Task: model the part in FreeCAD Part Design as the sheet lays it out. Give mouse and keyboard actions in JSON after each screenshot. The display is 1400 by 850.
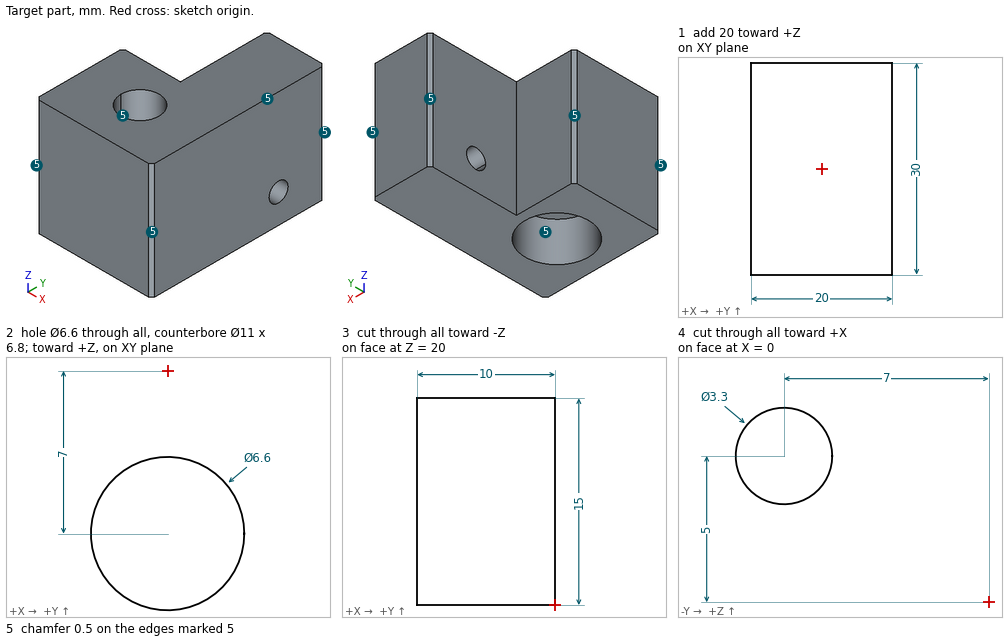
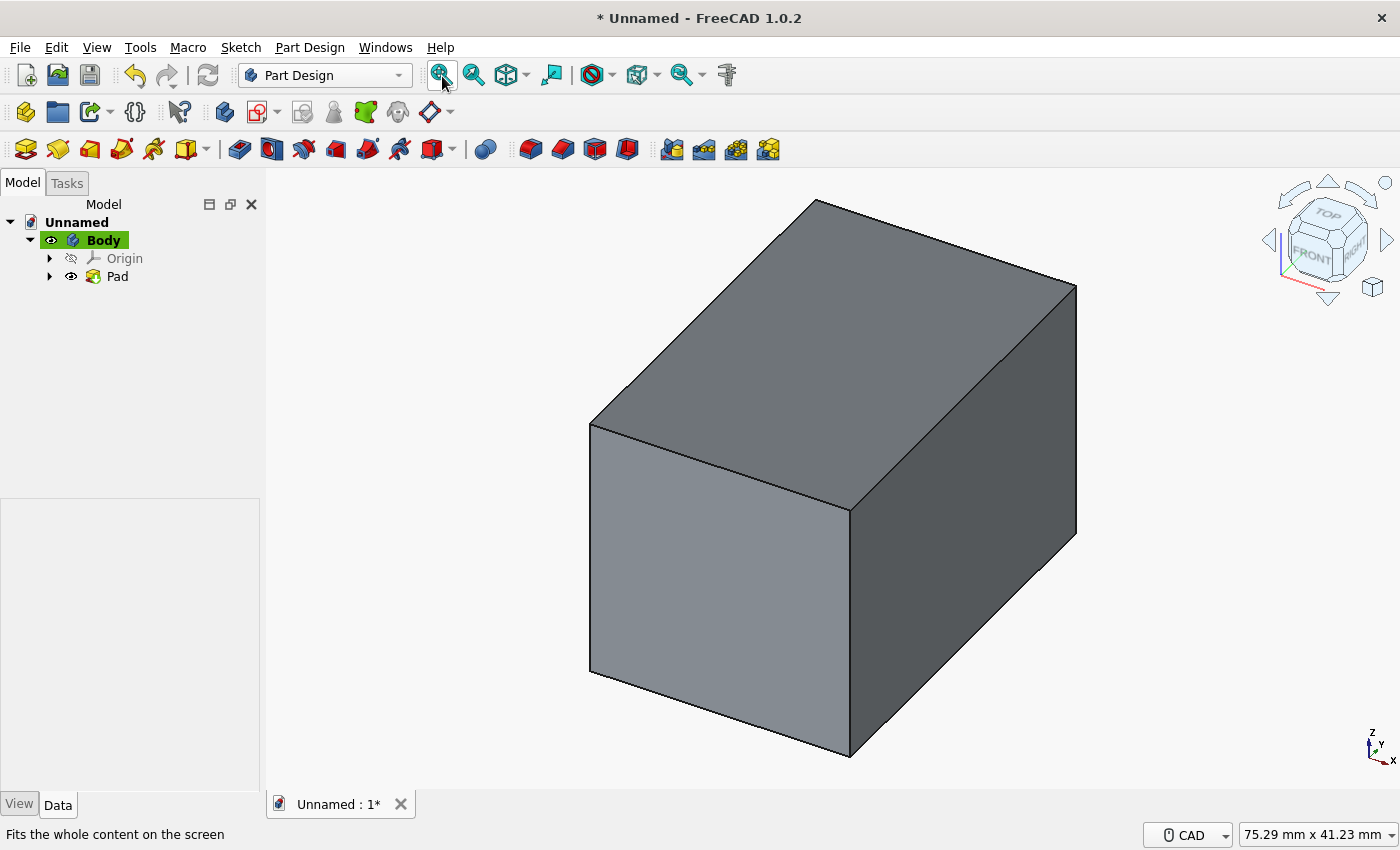
{"action": "left_click", "coordinate": [258, 112]}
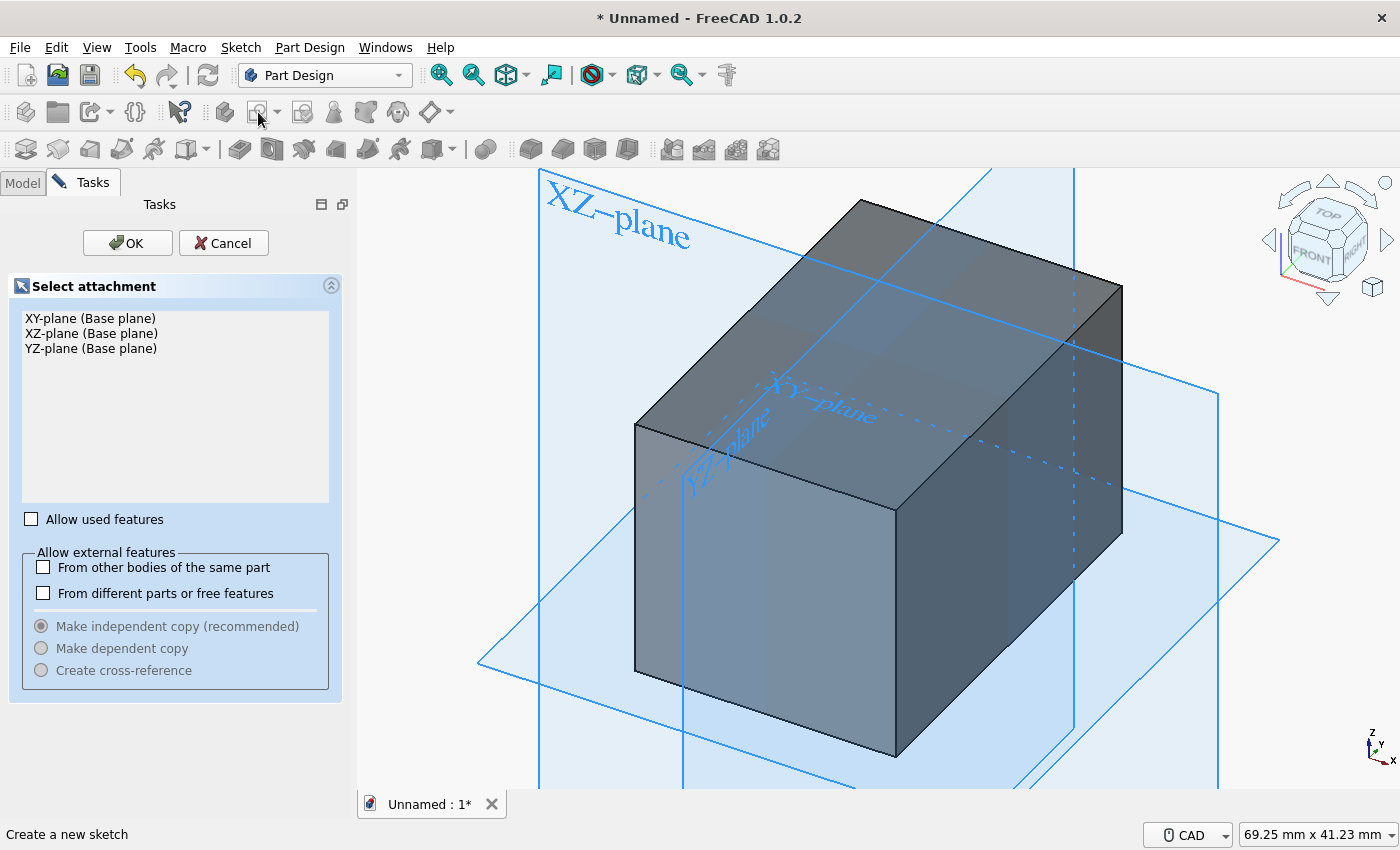
{"action": "left_click", "coordinate": [82, 318]}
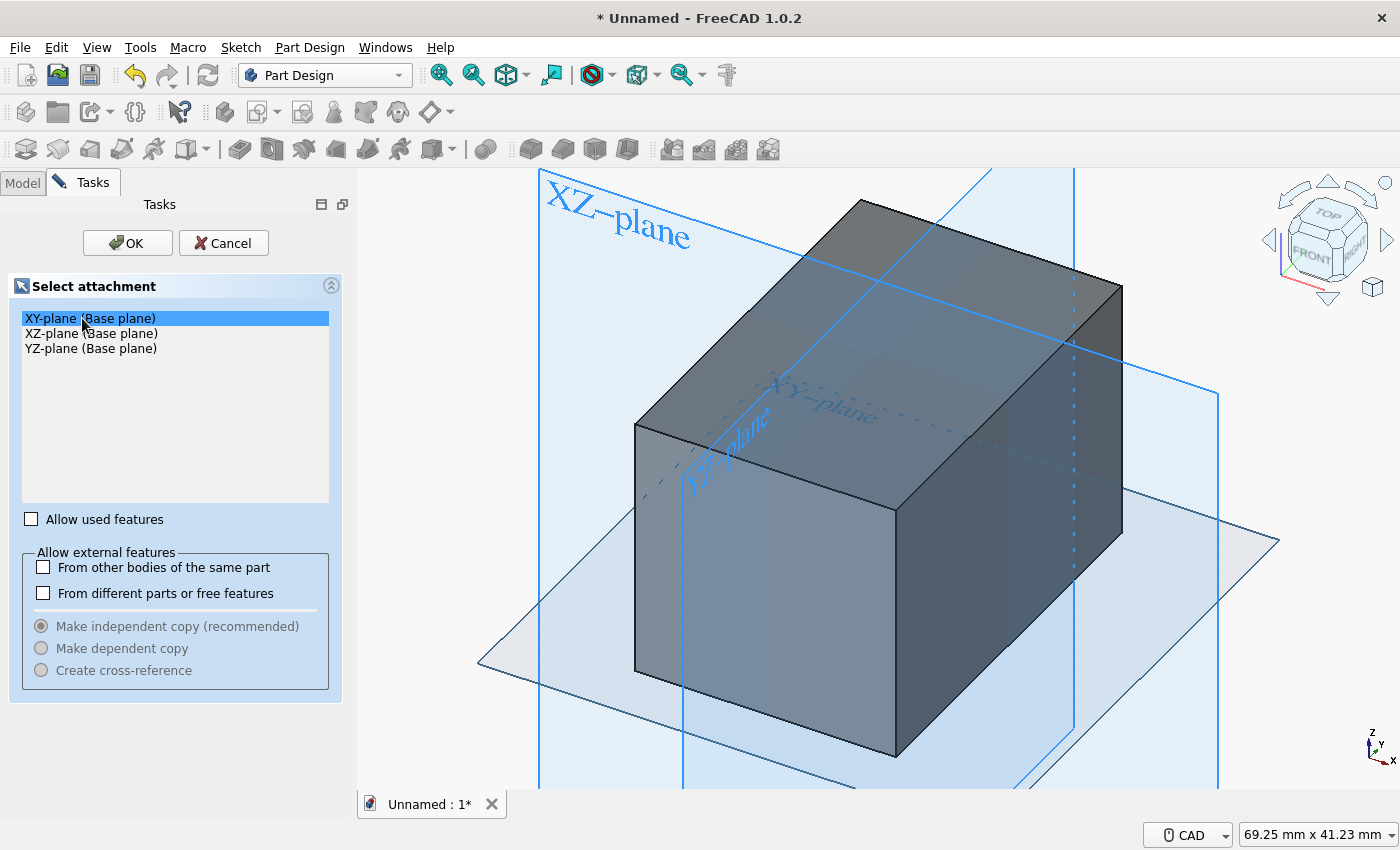
{"action": "left_click", "coordinate": [128, 243]}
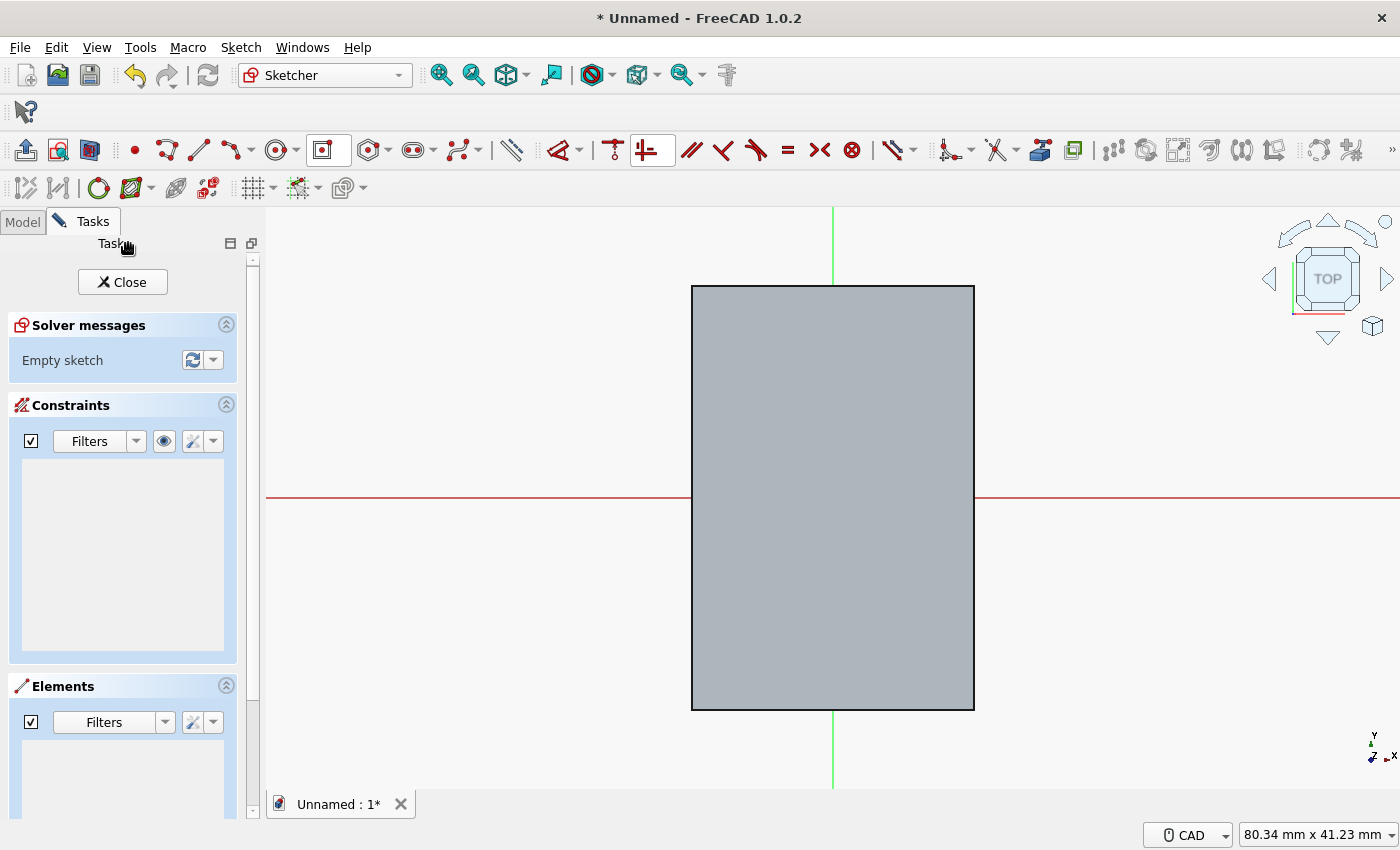
{"action": "key", "text": "q s"}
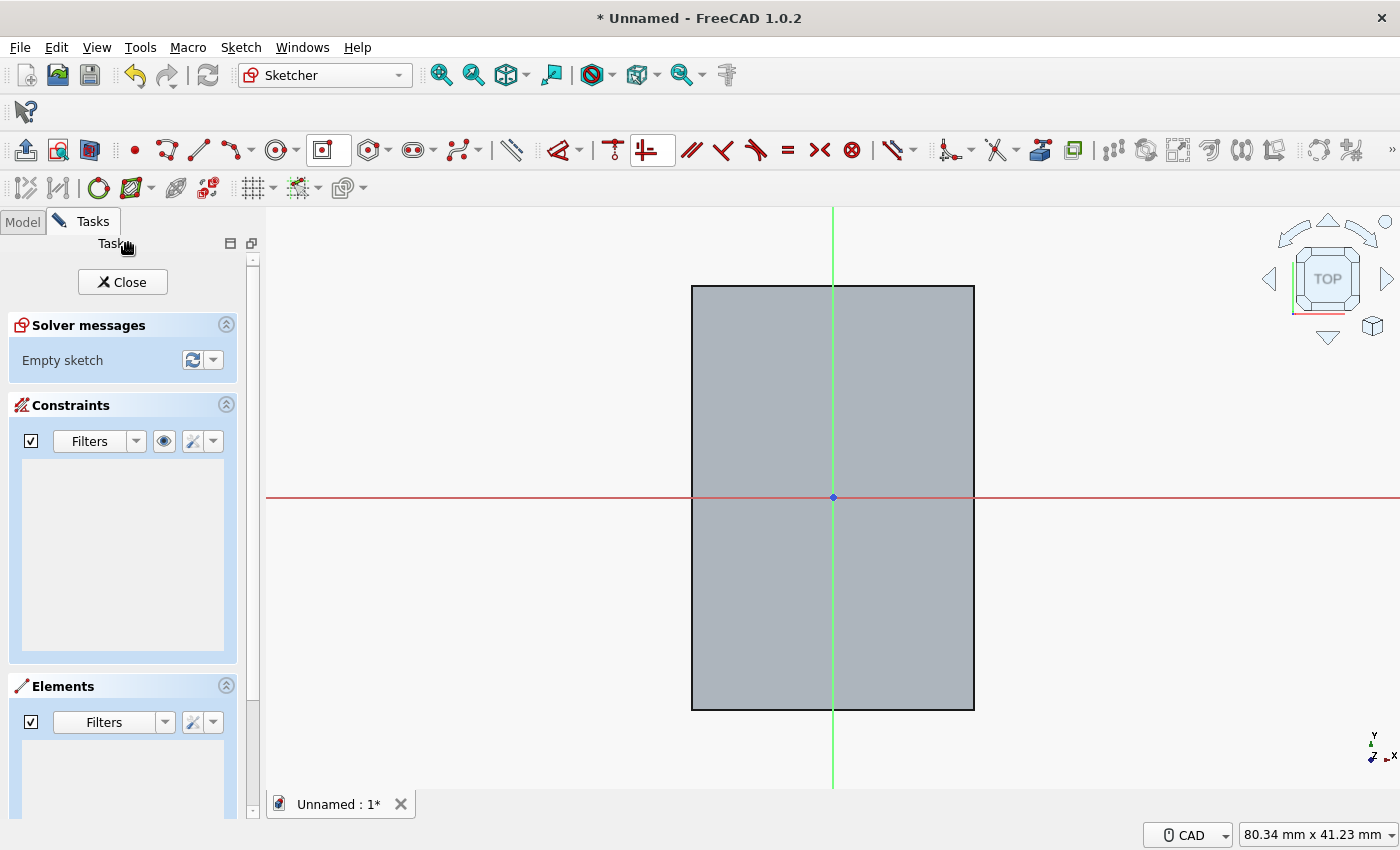
{"action": "scroll", "coordinate": [873, 613], "scroll_direction": "up", "scroll_amount": 5}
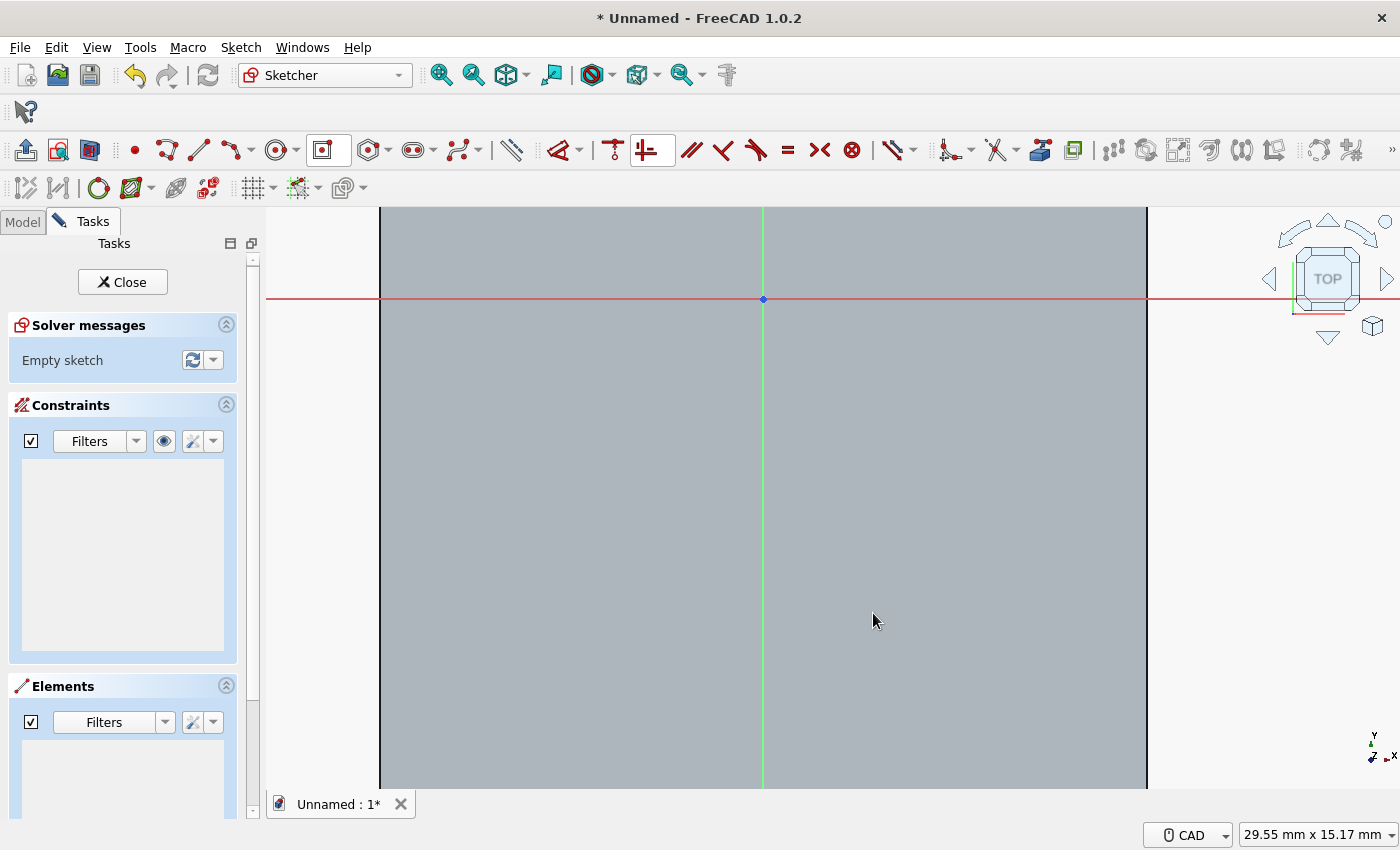
{"action": "key", "text": "g c"}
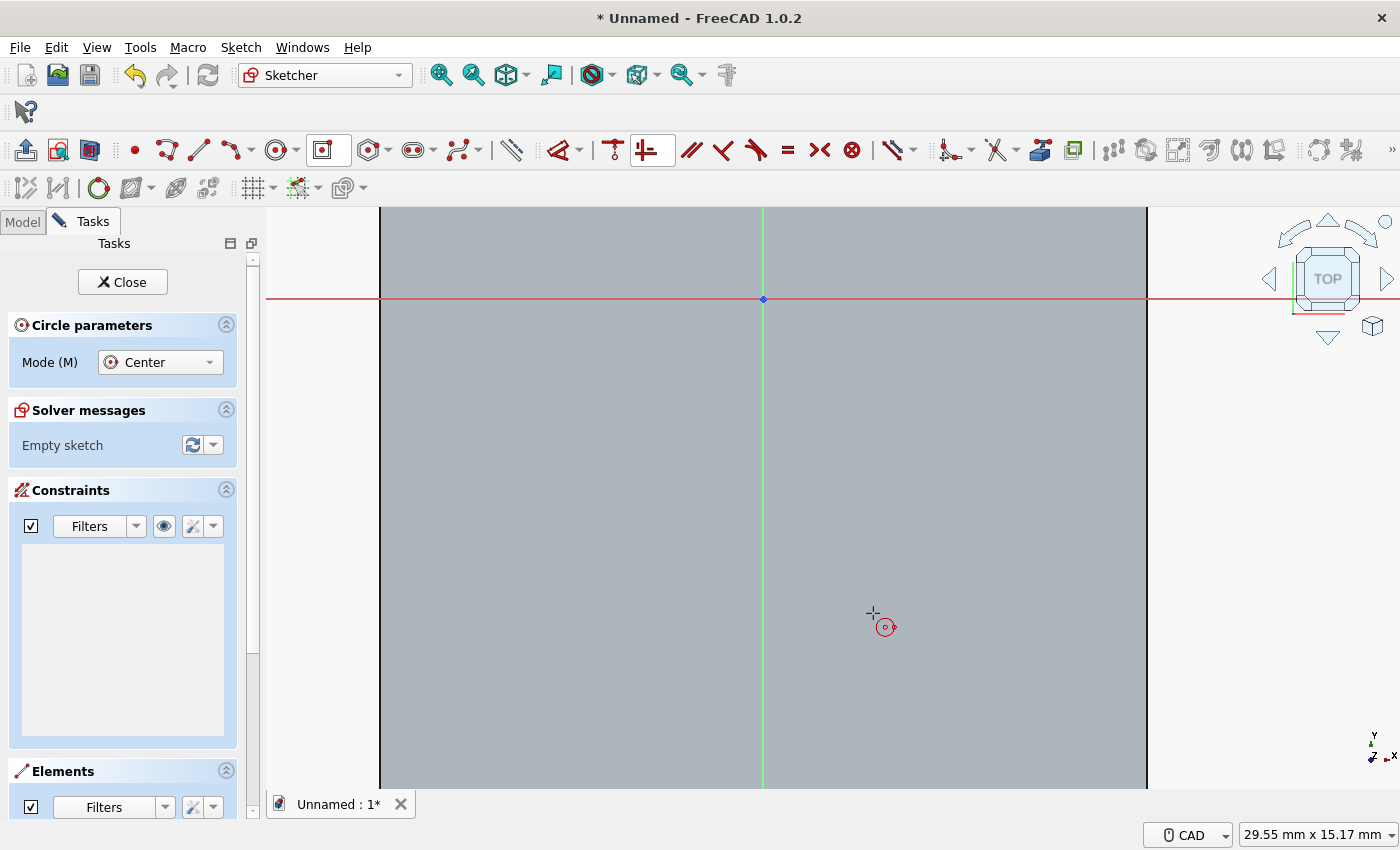
{"action": "left_click", "coordinate": [763, 568]}
{"action": "left_click", "coordinate": [853, 478]}
{"action": "key", "text": "Escape"}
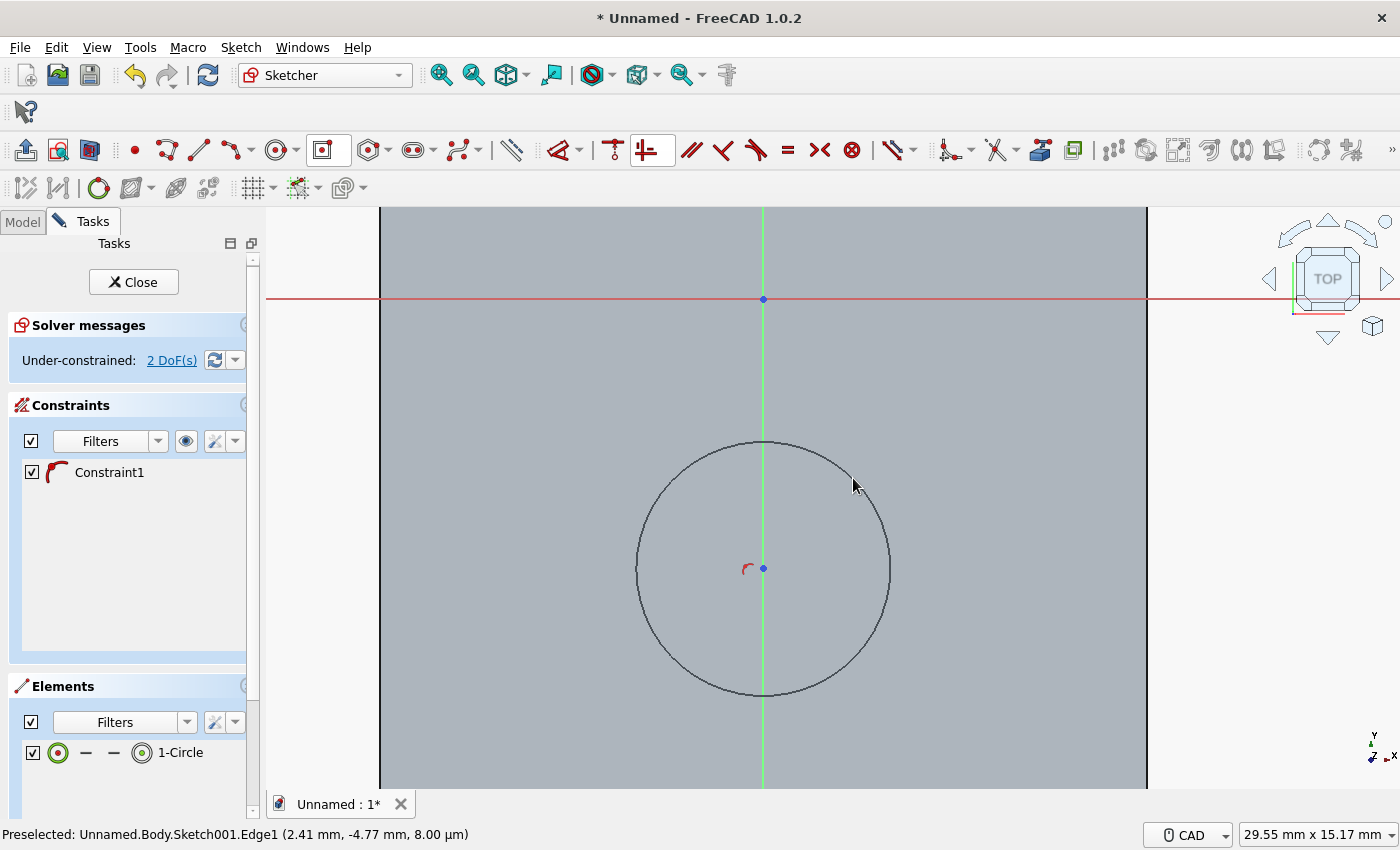
{"action": "left_click", "coordinate": [558, 150]}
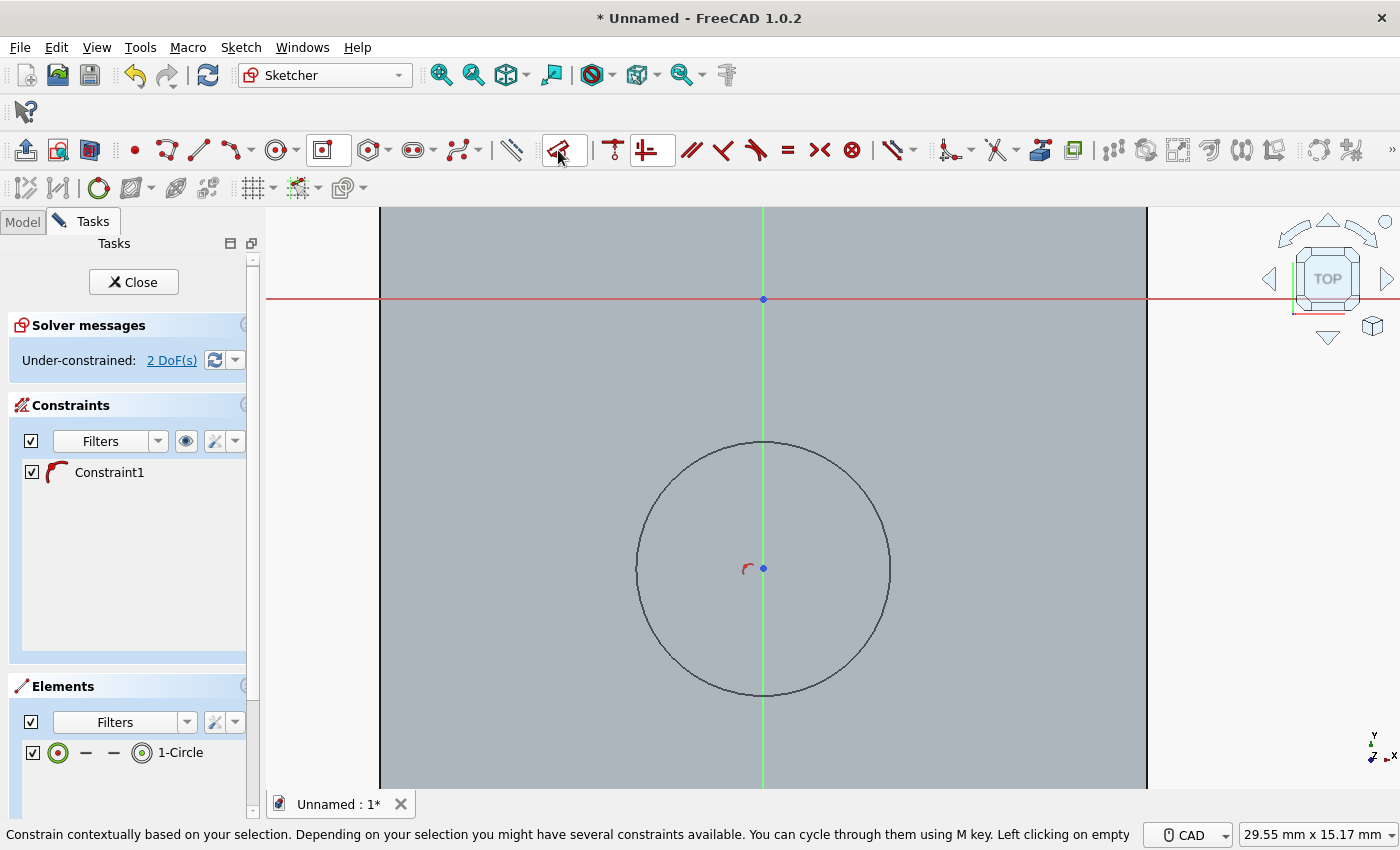
{"action": "left_click", "coordinate": [853, 479]}
{"action": "left_click", "coordinate": [876, 456]}